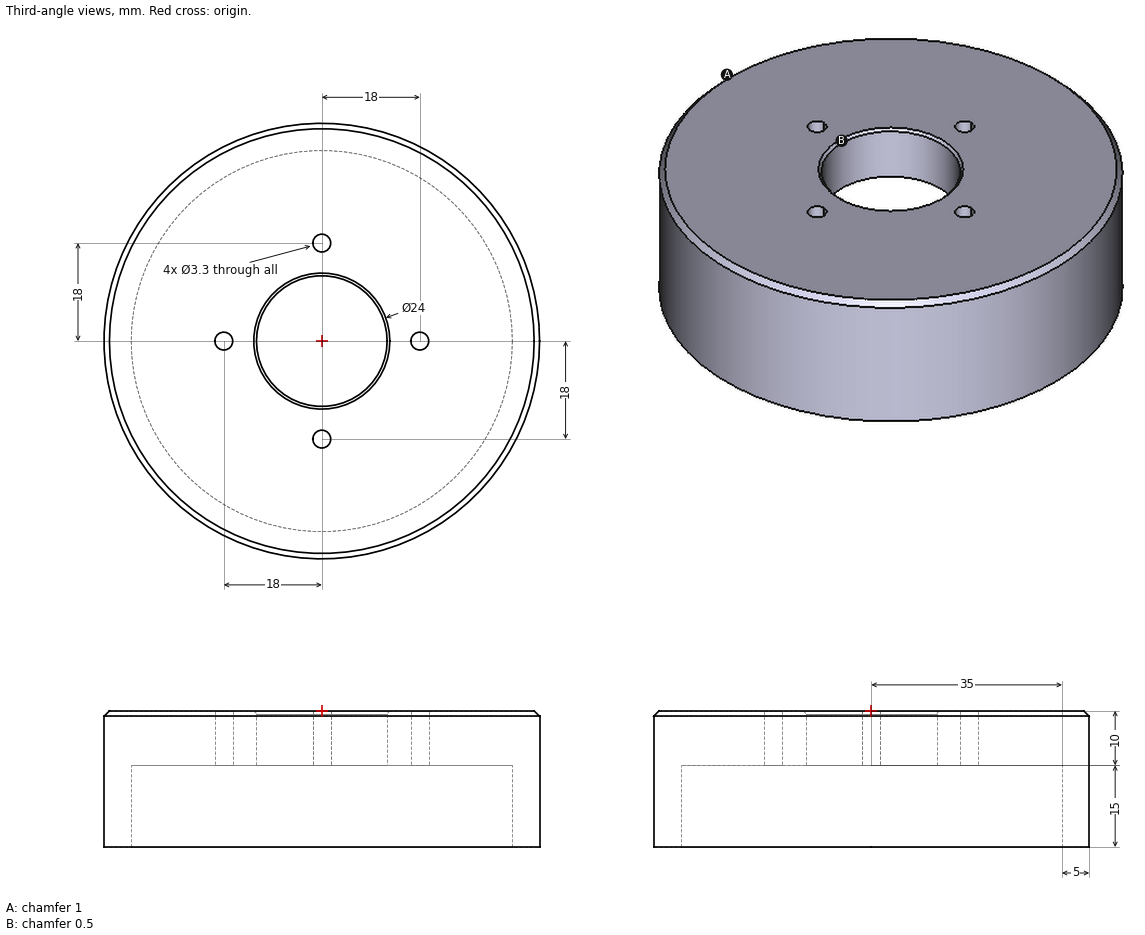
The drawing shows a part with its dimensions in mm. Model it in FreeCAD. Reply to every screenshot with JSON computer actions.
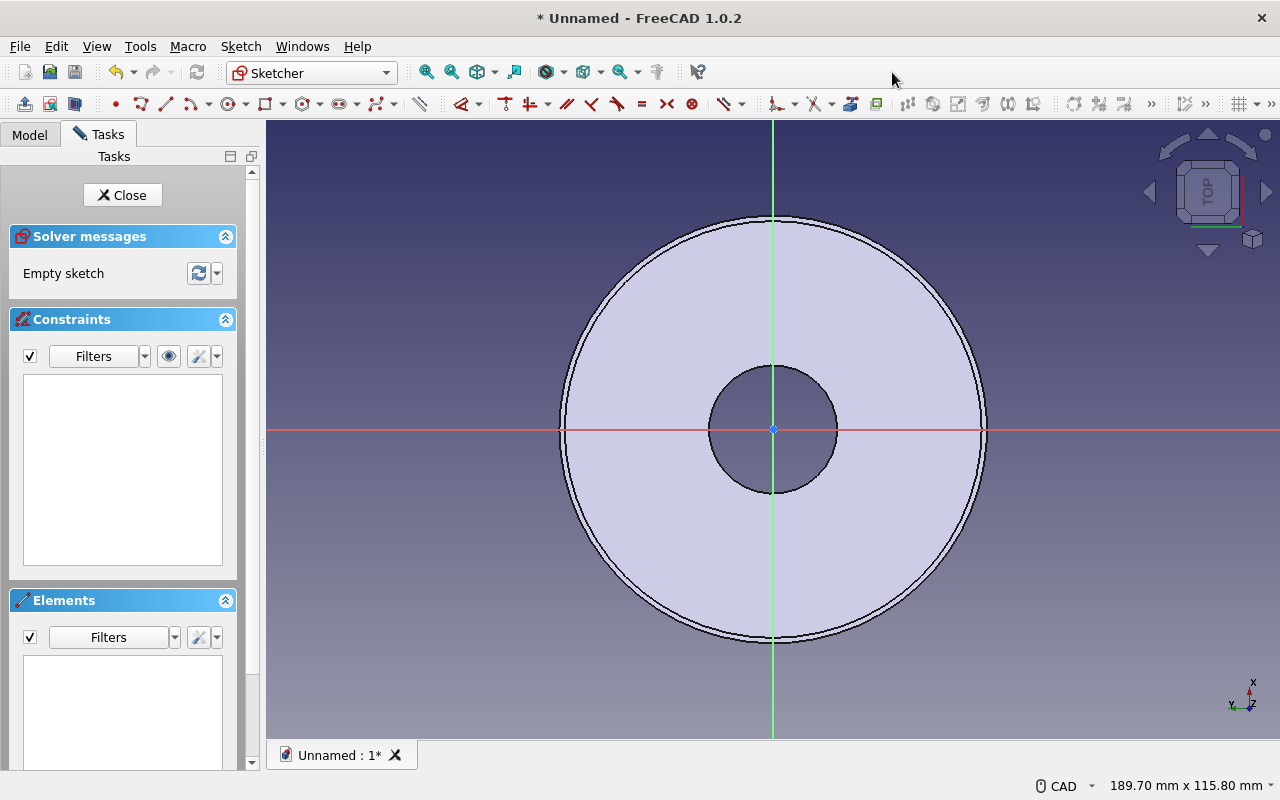
{"action": "scroll", "coordinate": [857, 430], "scroll_direction": "up", "scroll_amount": 3}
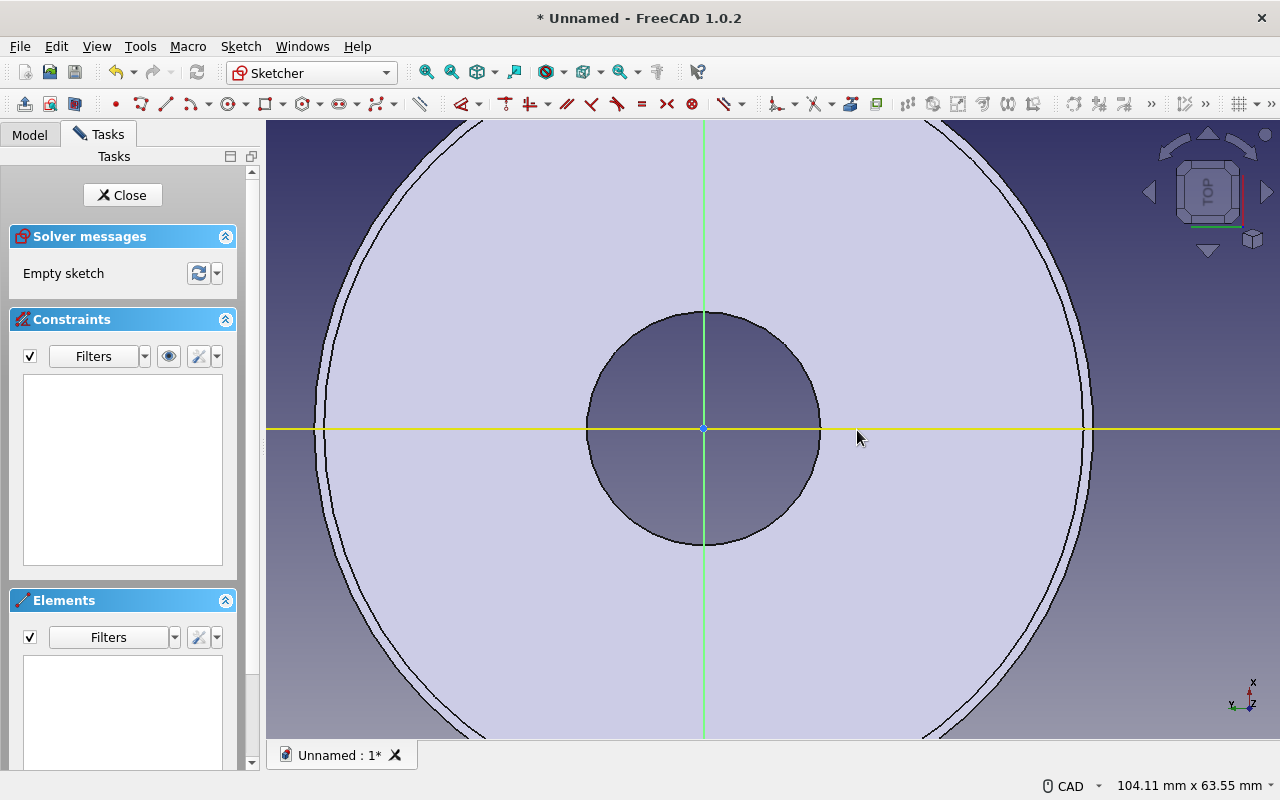
{"action": "left_click", "coordinate": [228, 104]}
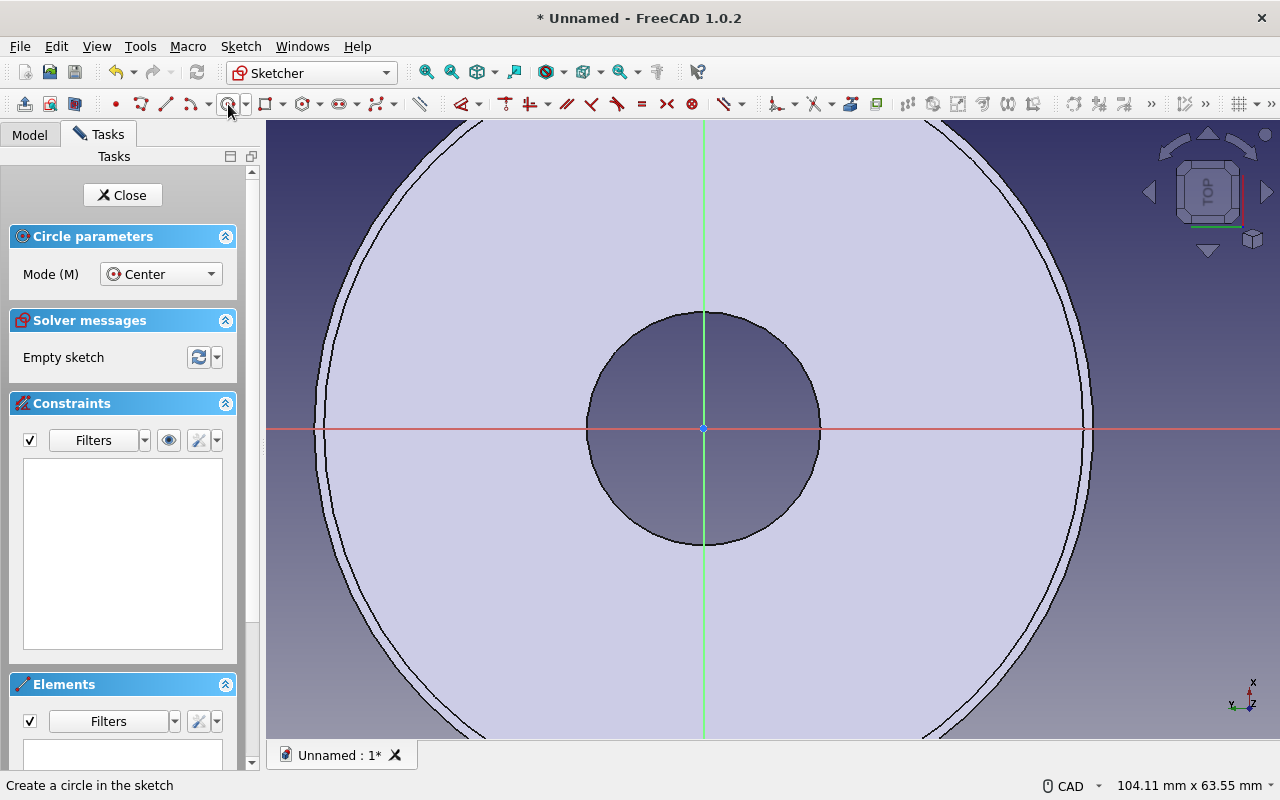
{"action": "scroll", "coordinate": [528, 429], "scroll_direction": "up", "scroll_amount": 2}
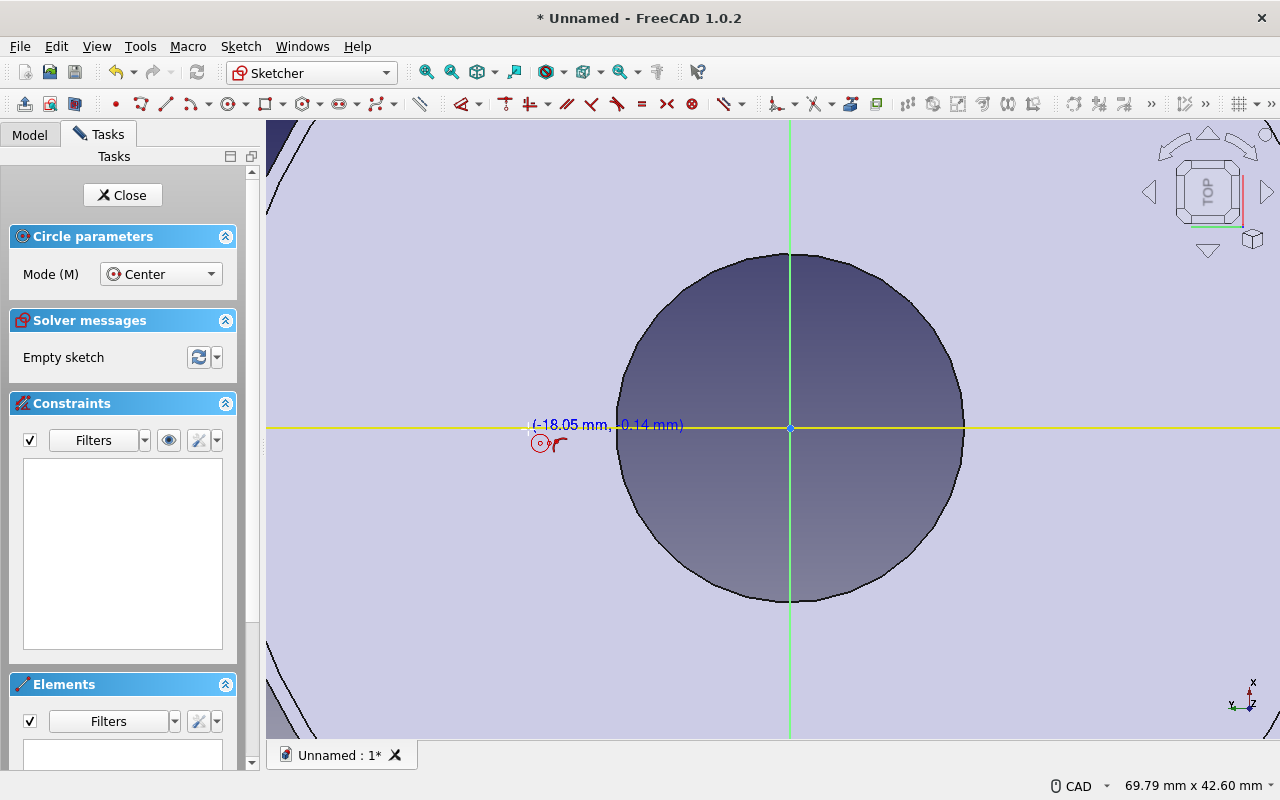
{"action": "left_click", "coordinate": [529, 428]}
{"action": "mouse_move", "coordinate": [545, 411]}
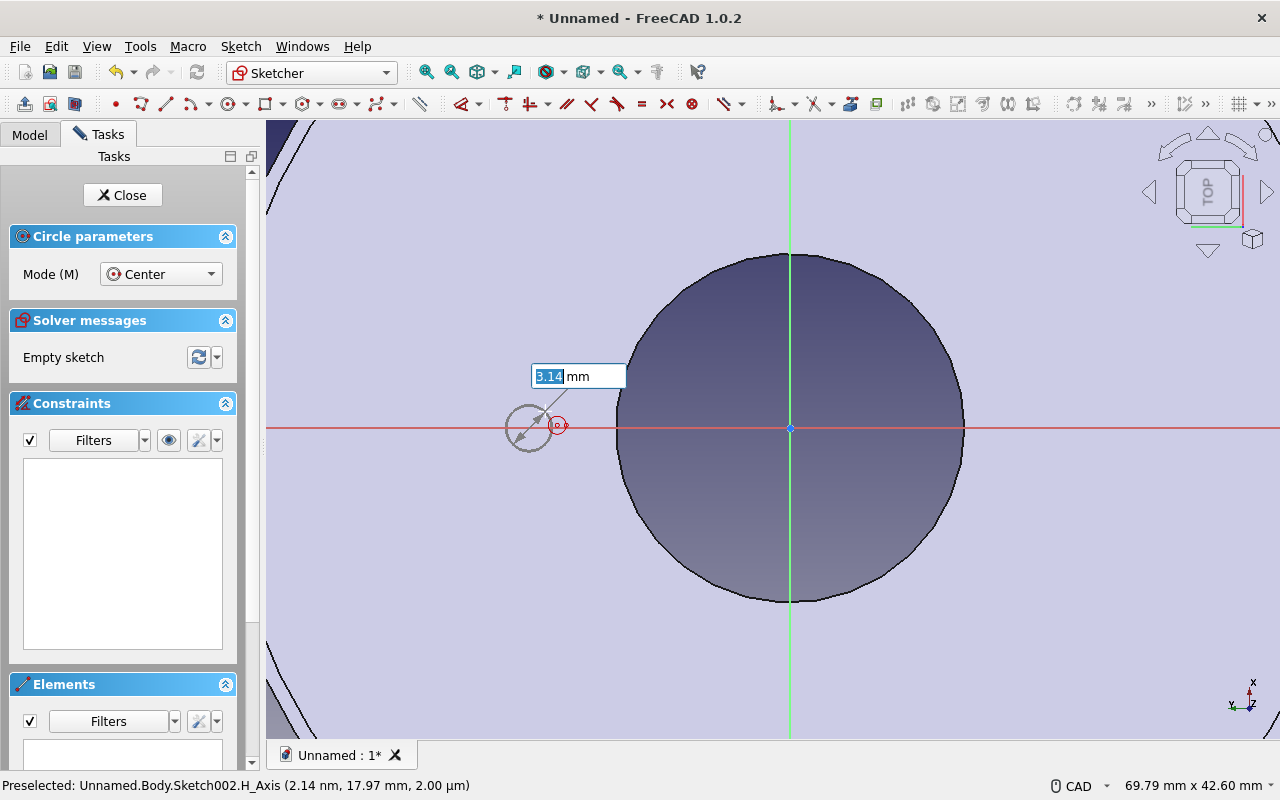
{"action": "type", "text": "3.3"}
{"action": "key", "text": "Return"}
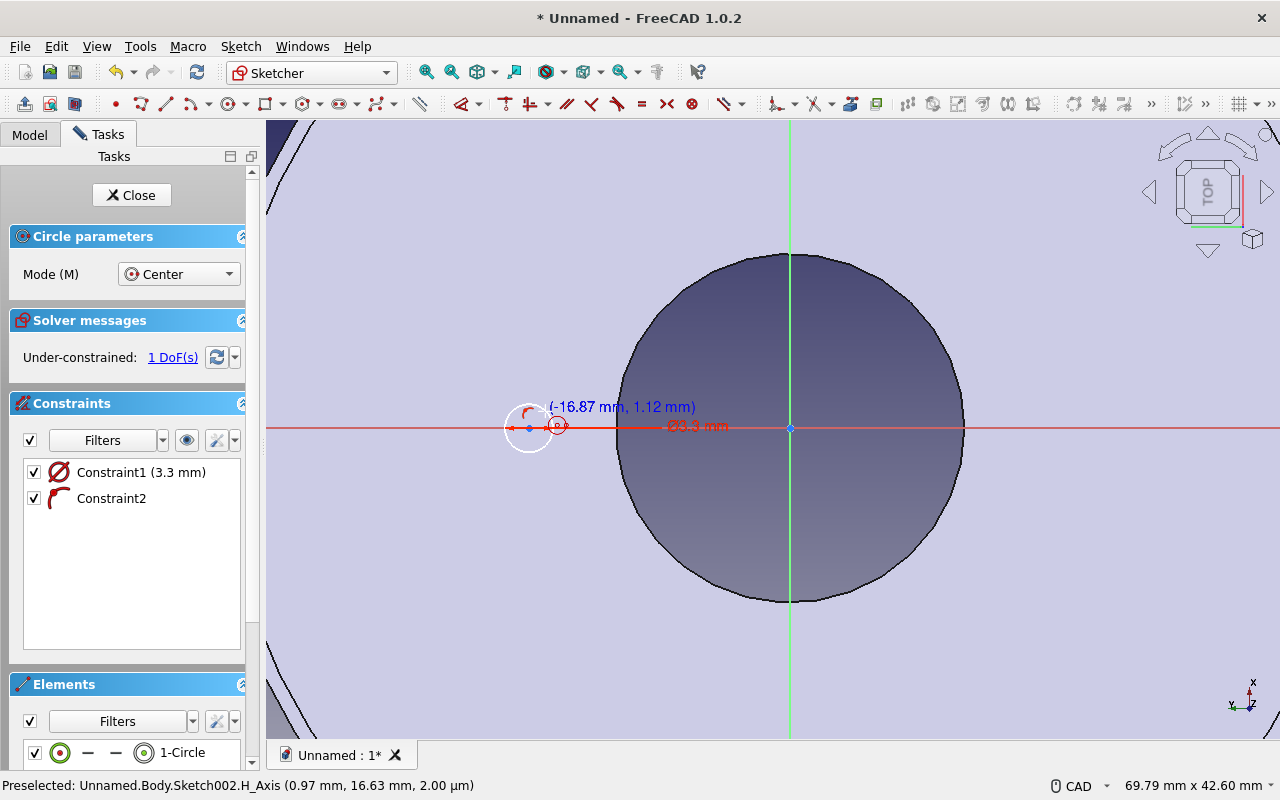
{"action": "left_click", "coordinate": [790, 690]}
{"action": "mouse_move", "coordinate": [807, 673]}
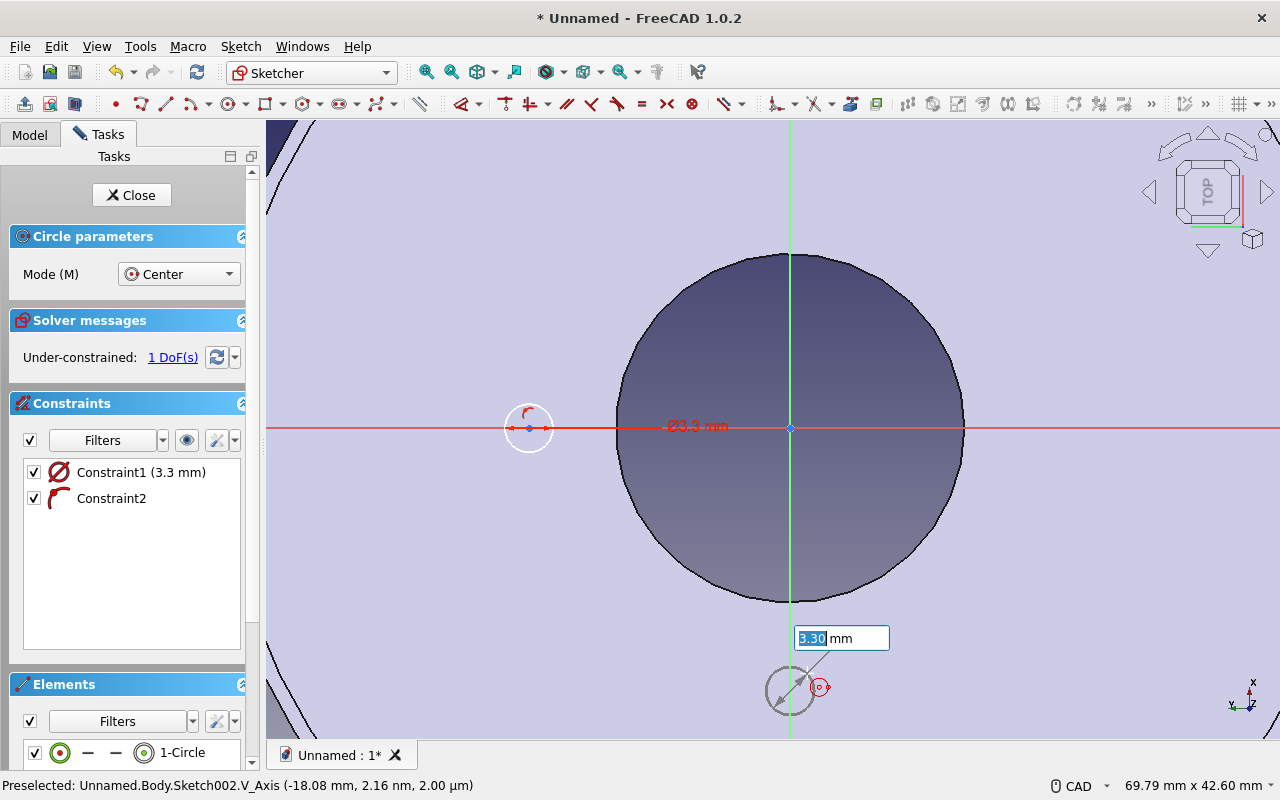
{"action": "type", "text": "3.3"}
{"action": "key", "text": "Return"}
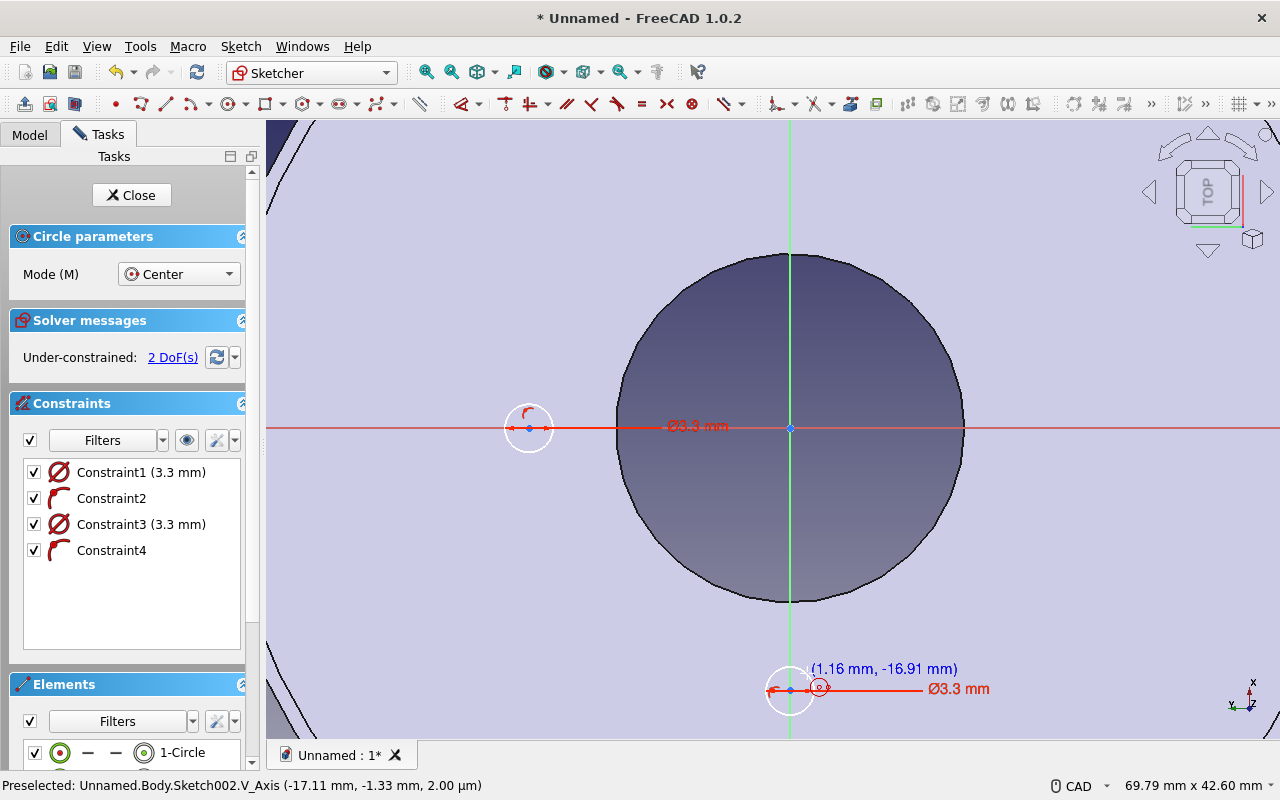
{"action": "left_click", "coordinate": [790, 167]}
{"action": "mouse_move", "coordinate": [807, 150]}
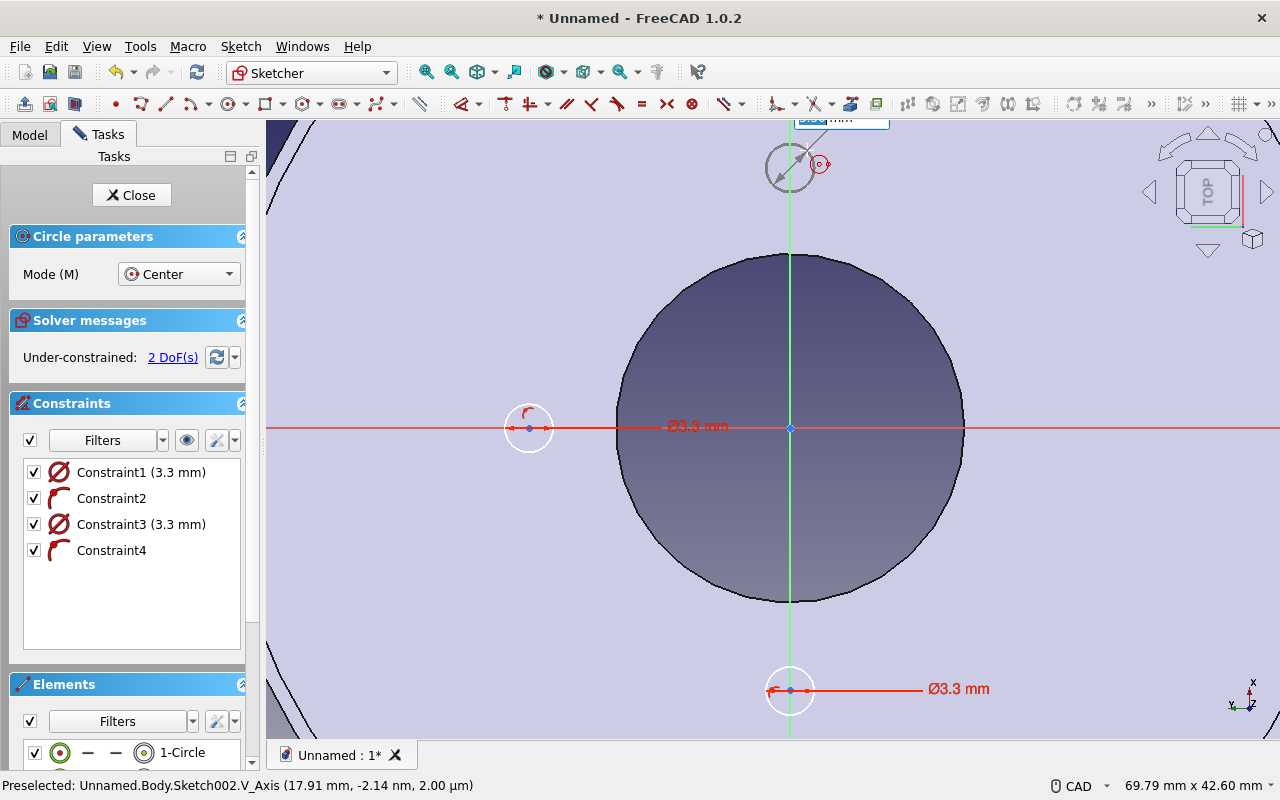
{"action": "type", "text": "3.3"}
{"action": "key", "text": "Return"}